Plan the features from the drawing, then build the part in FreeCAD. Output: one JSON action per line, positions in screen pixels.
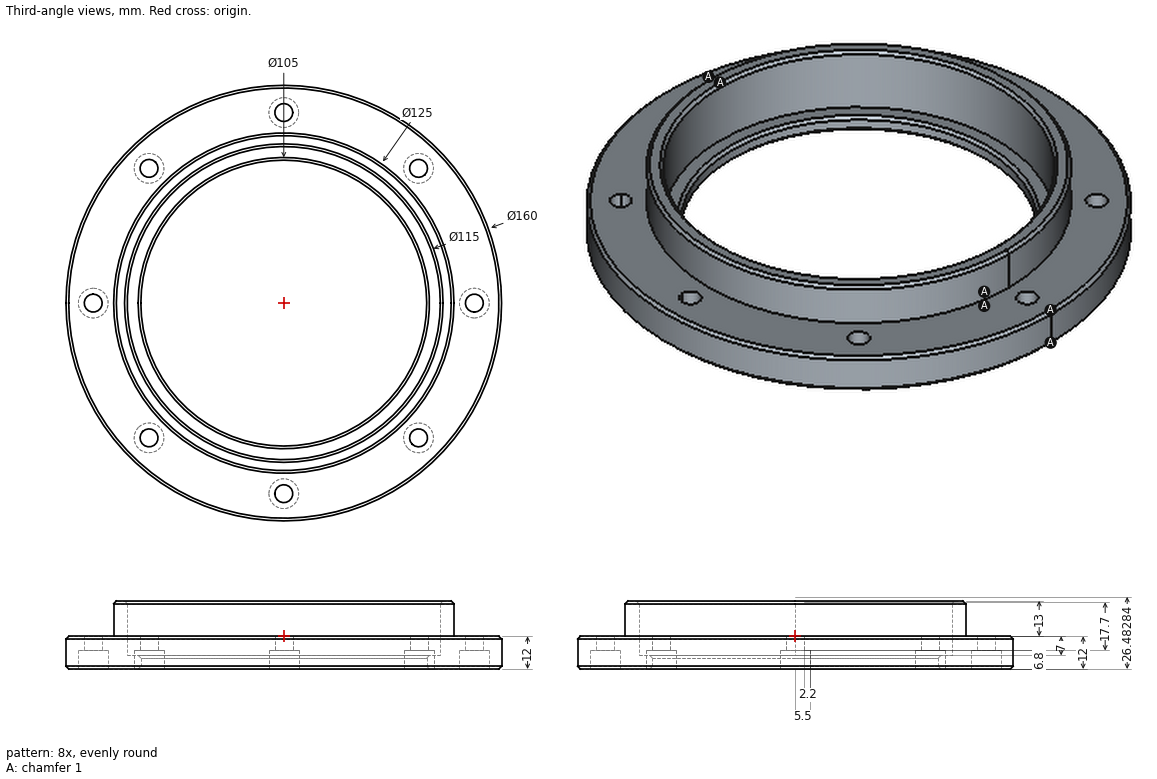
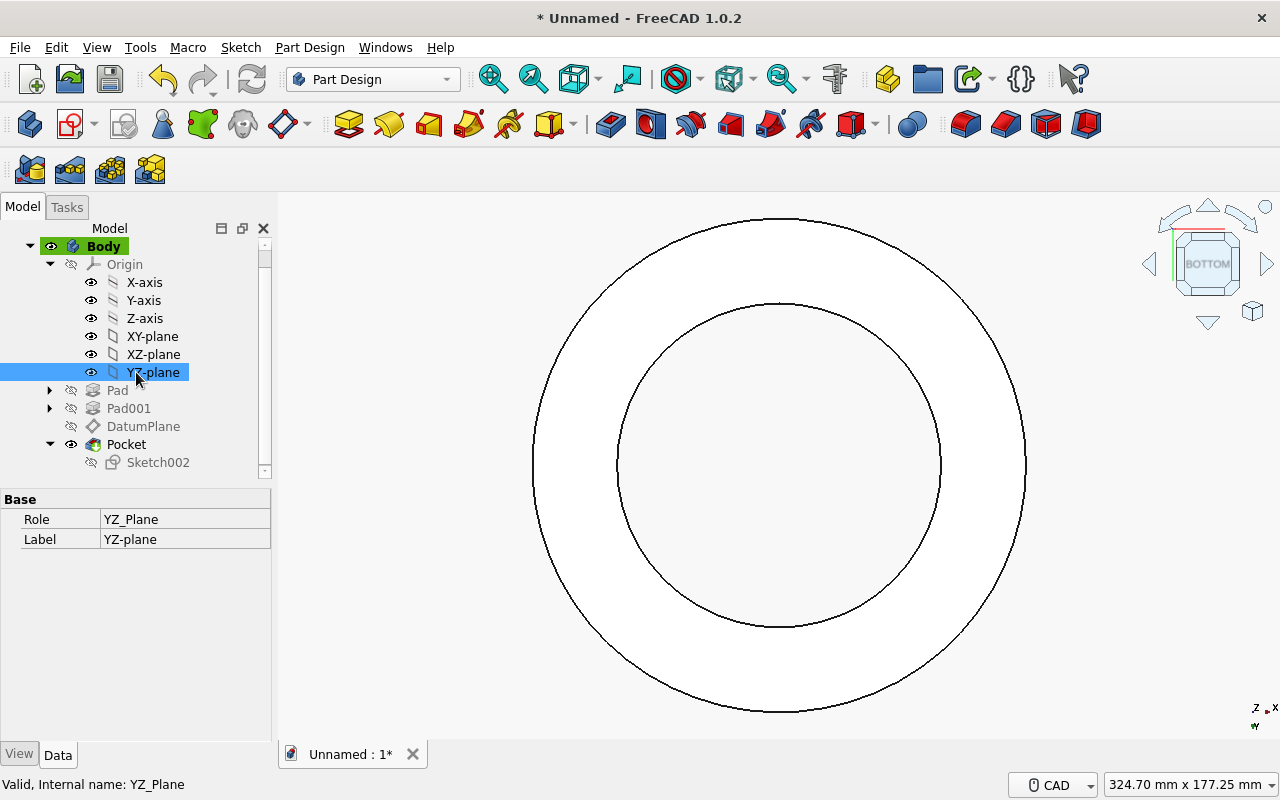
{"action": "left_click", "coordinate": [284, 124]}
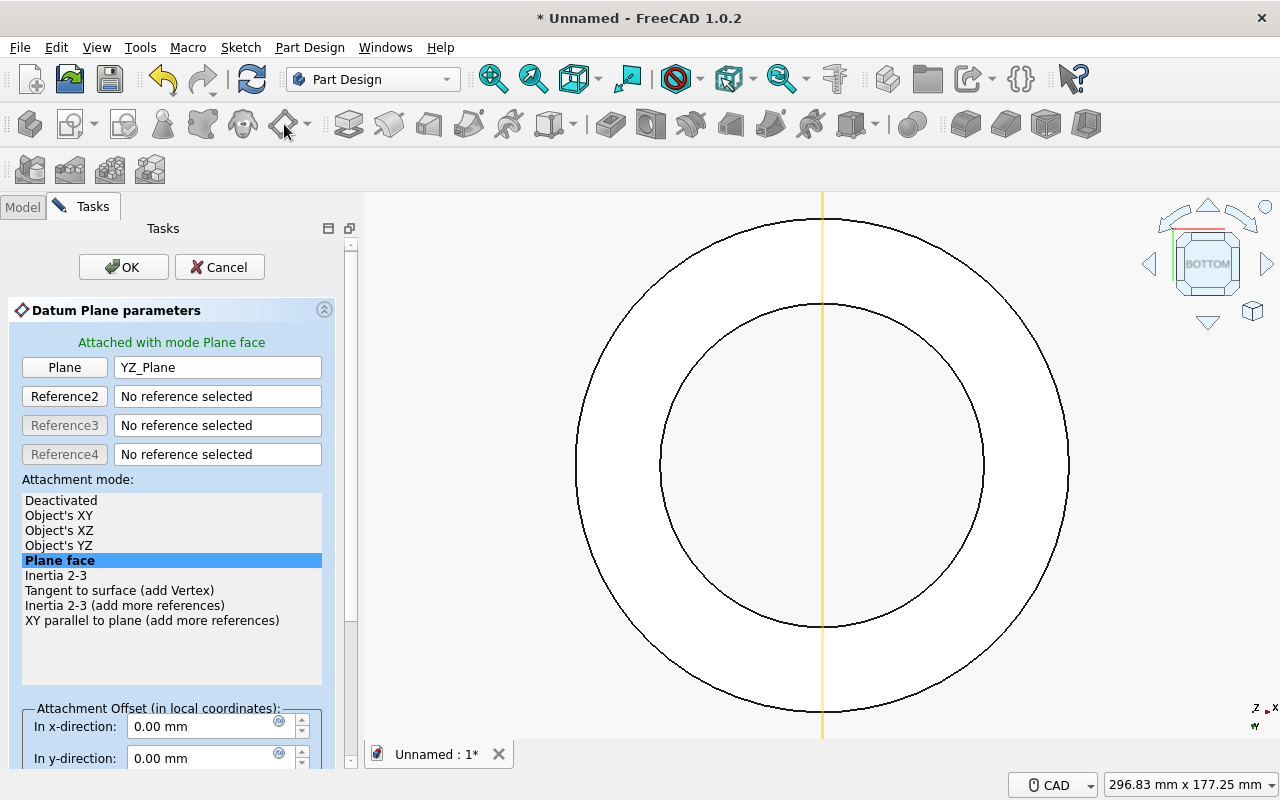
{"action": "scroll", "coordinate": [351, 503], "scroll_direction": "down", "scroll_amount": 2}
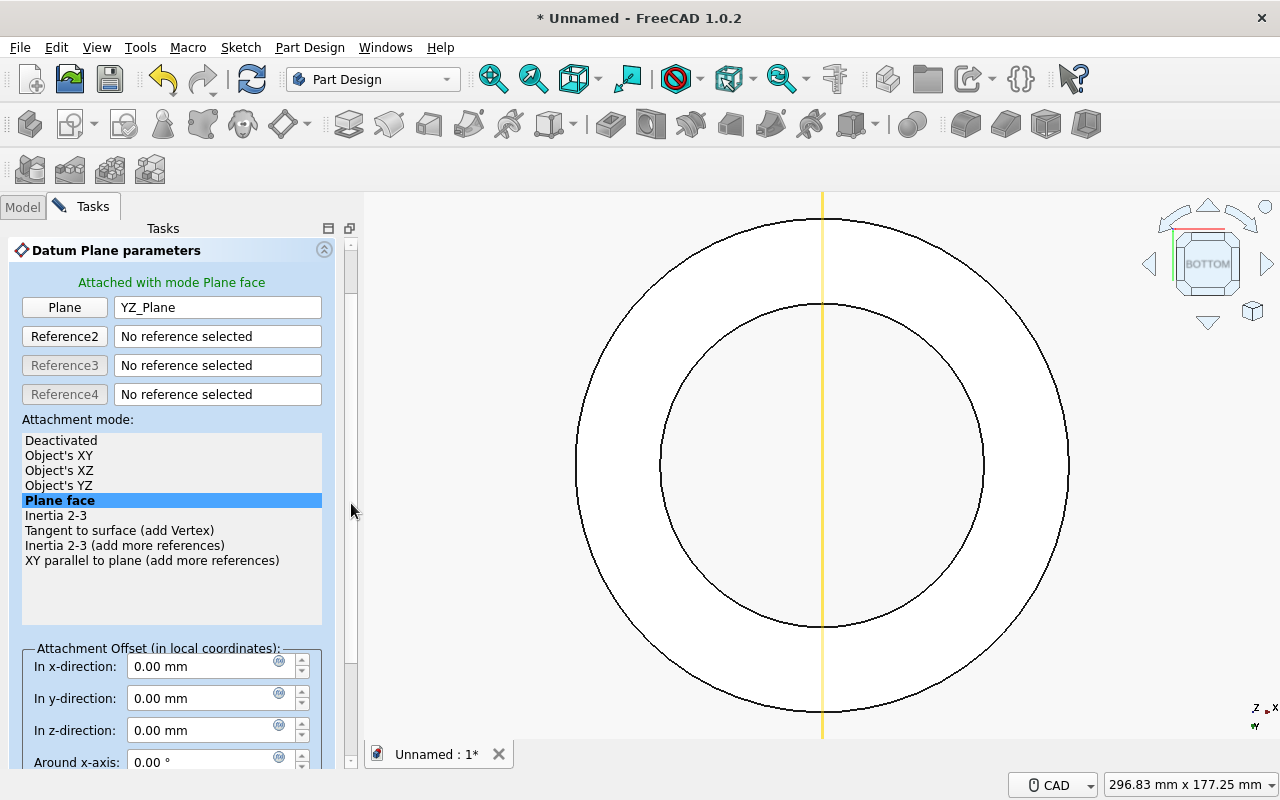
{"action": "triple_click", "coordinate": [210, 670]}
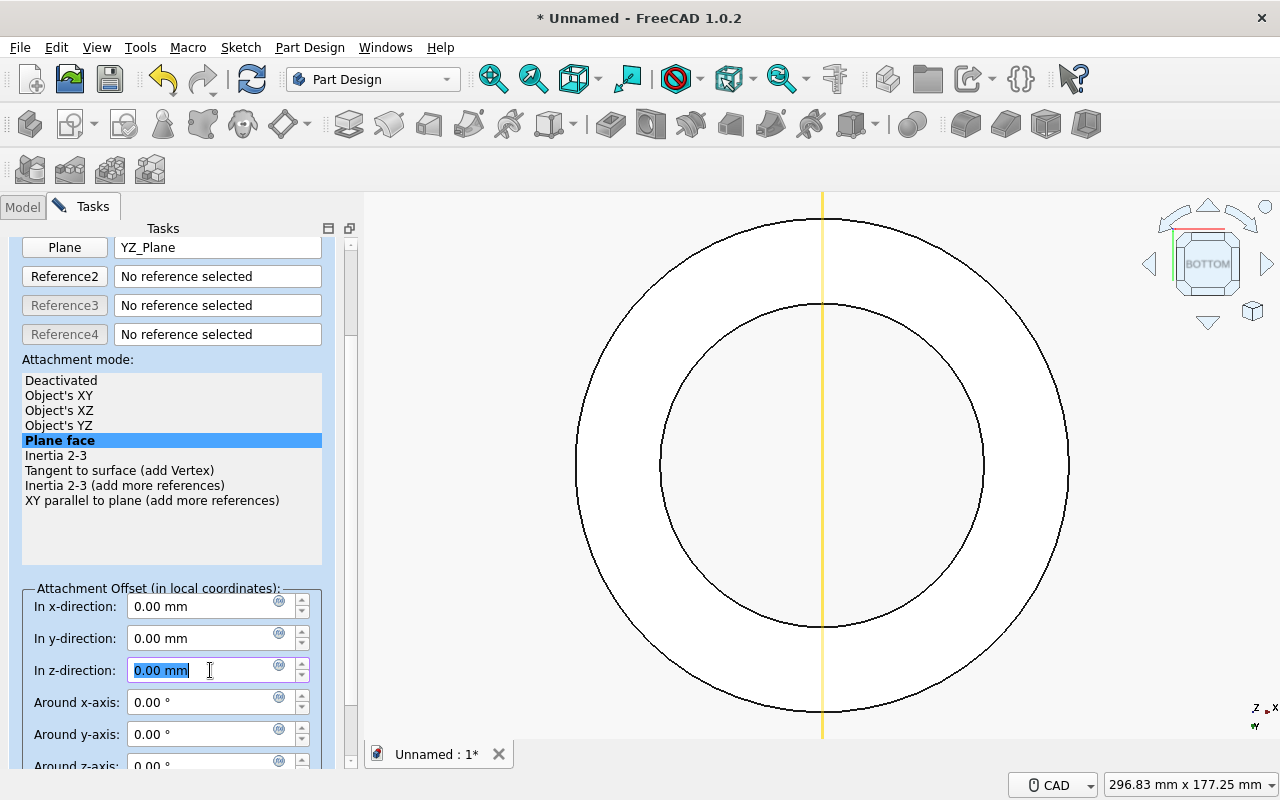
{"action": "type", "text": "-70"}
{"action": "key", "text": "Tab"}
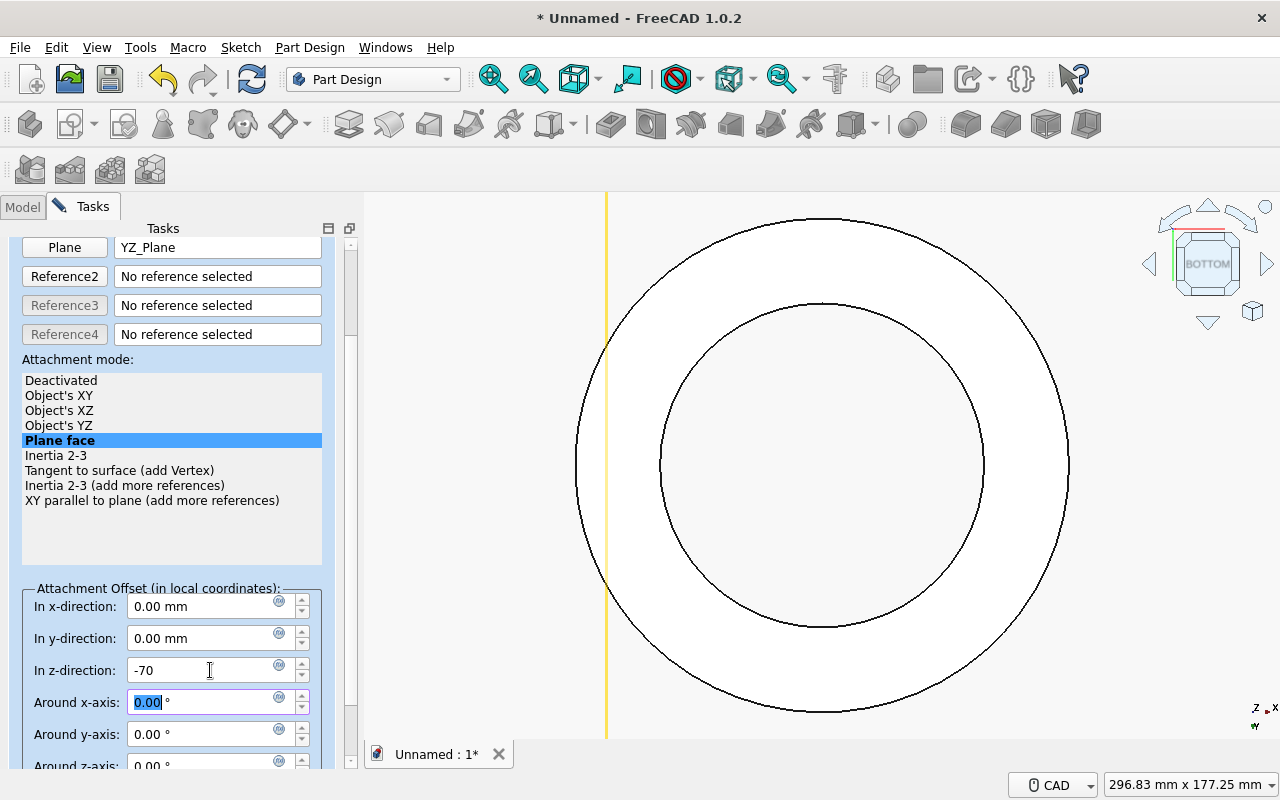
{"action": "scroll", "coordinate": [351, 503], "scroll_direction": "up", "scroll_amount": 3}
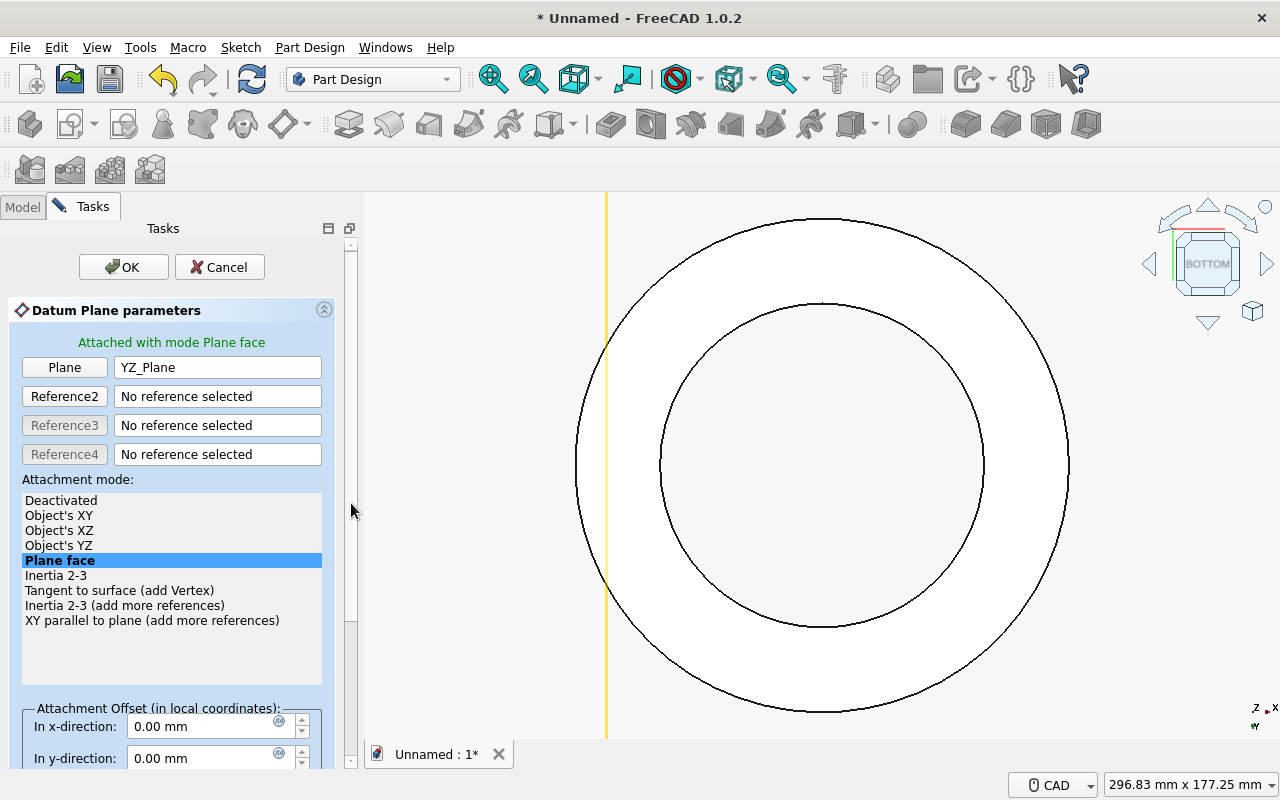
{"action": "left_click", "coordinate": [124, 267]}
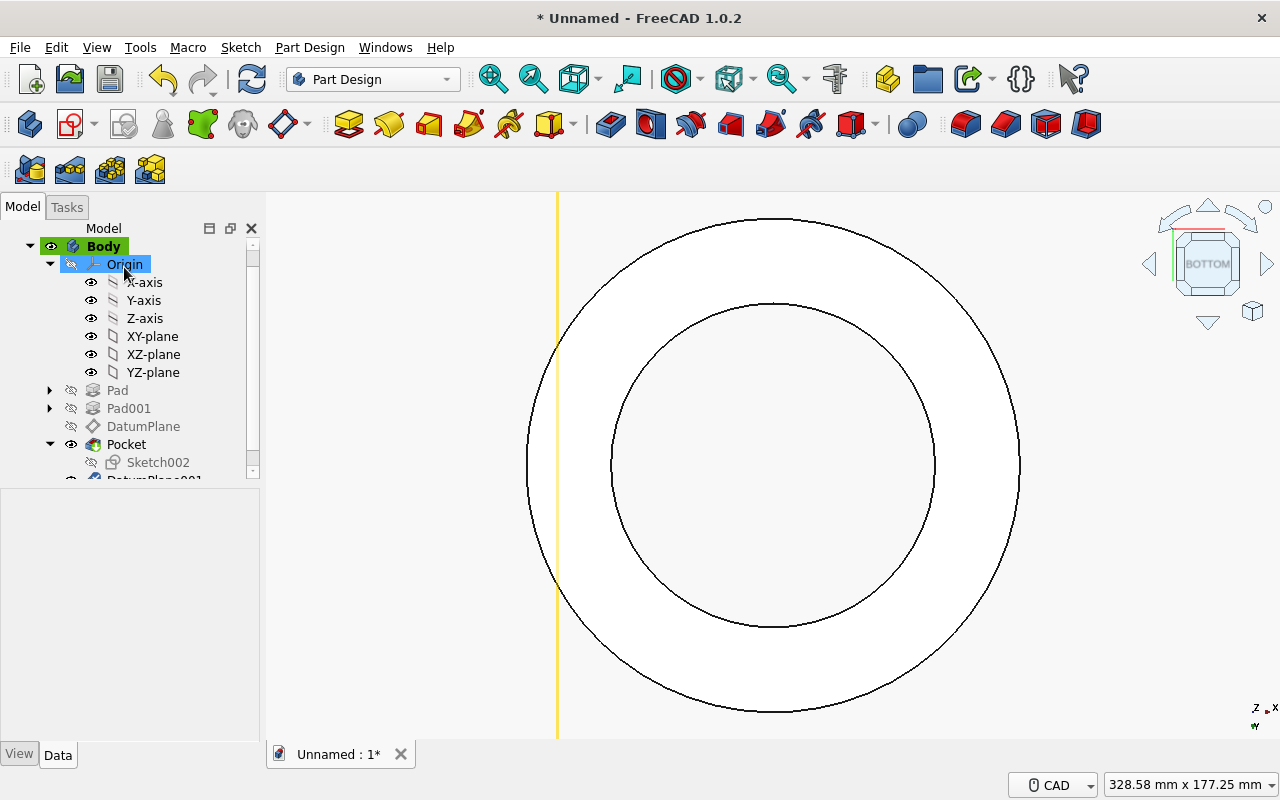
{"action": "scroll", "coordinate": [120, 350], "scroll_direction": "down", "scroll_amount": 3}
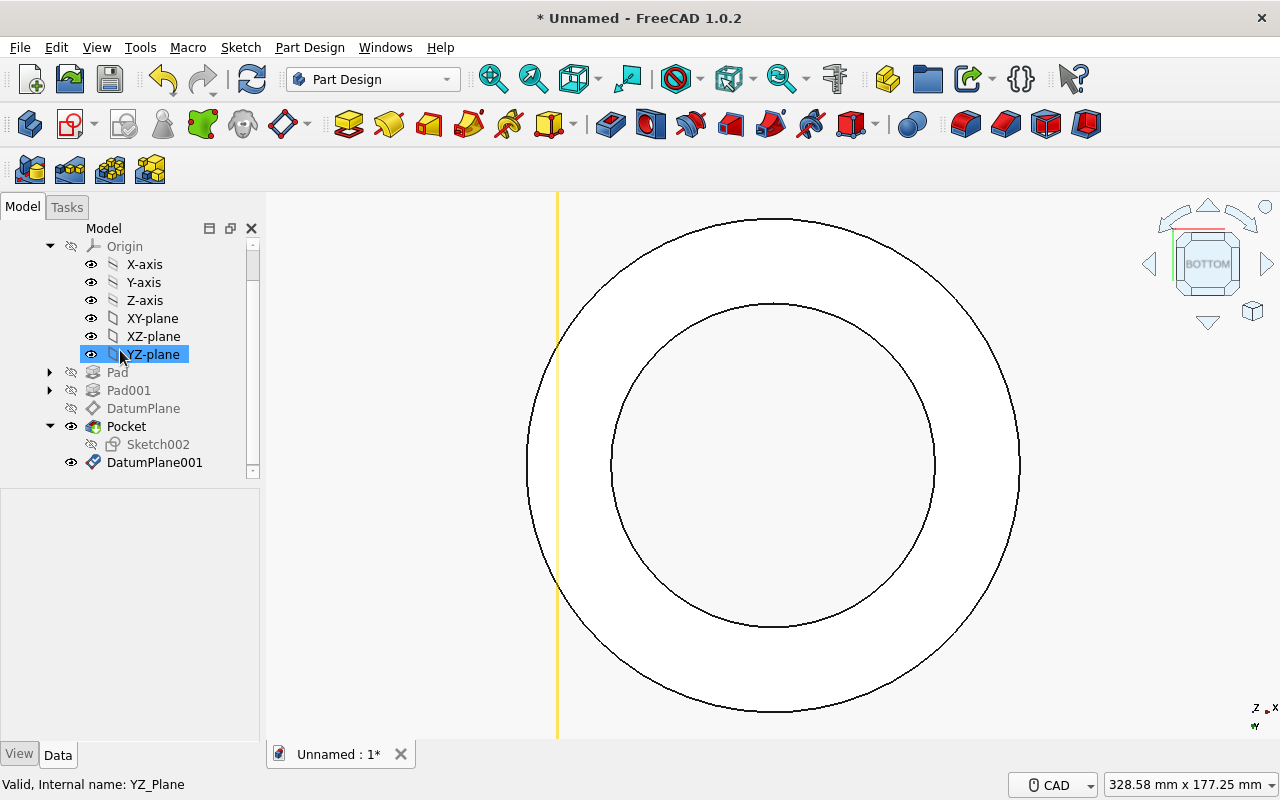
{"action": "left_click", "coordinate": [116, 462]}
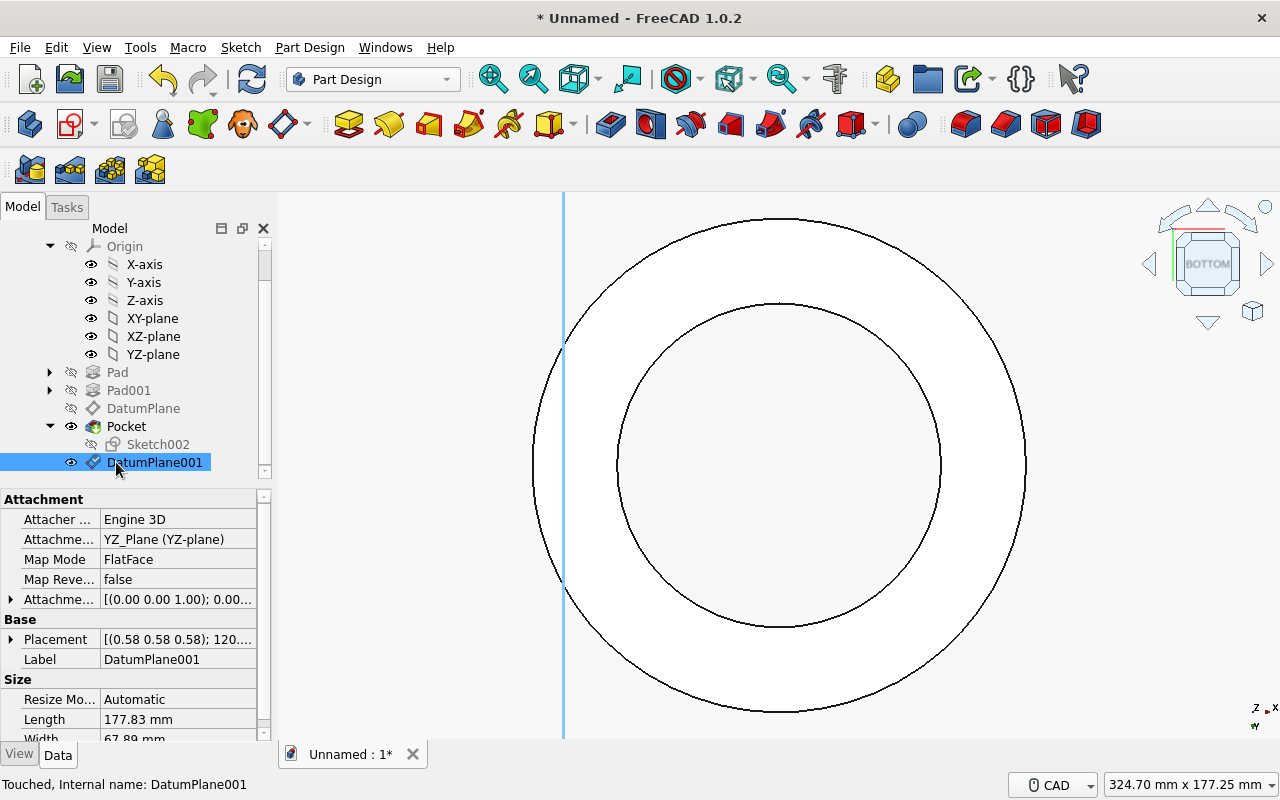
{"action": "left_click", "coordinate": [70, 124]}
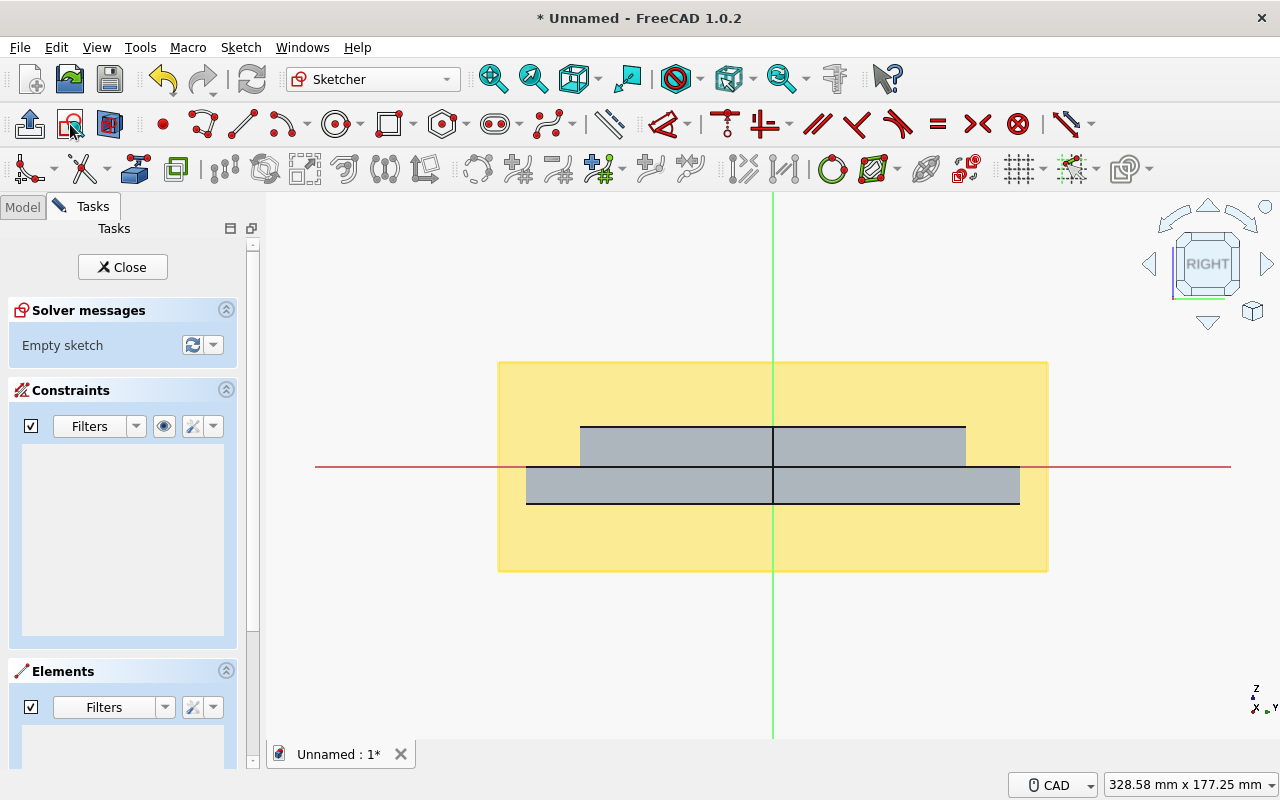
{"action": "key", "text": "q s"}